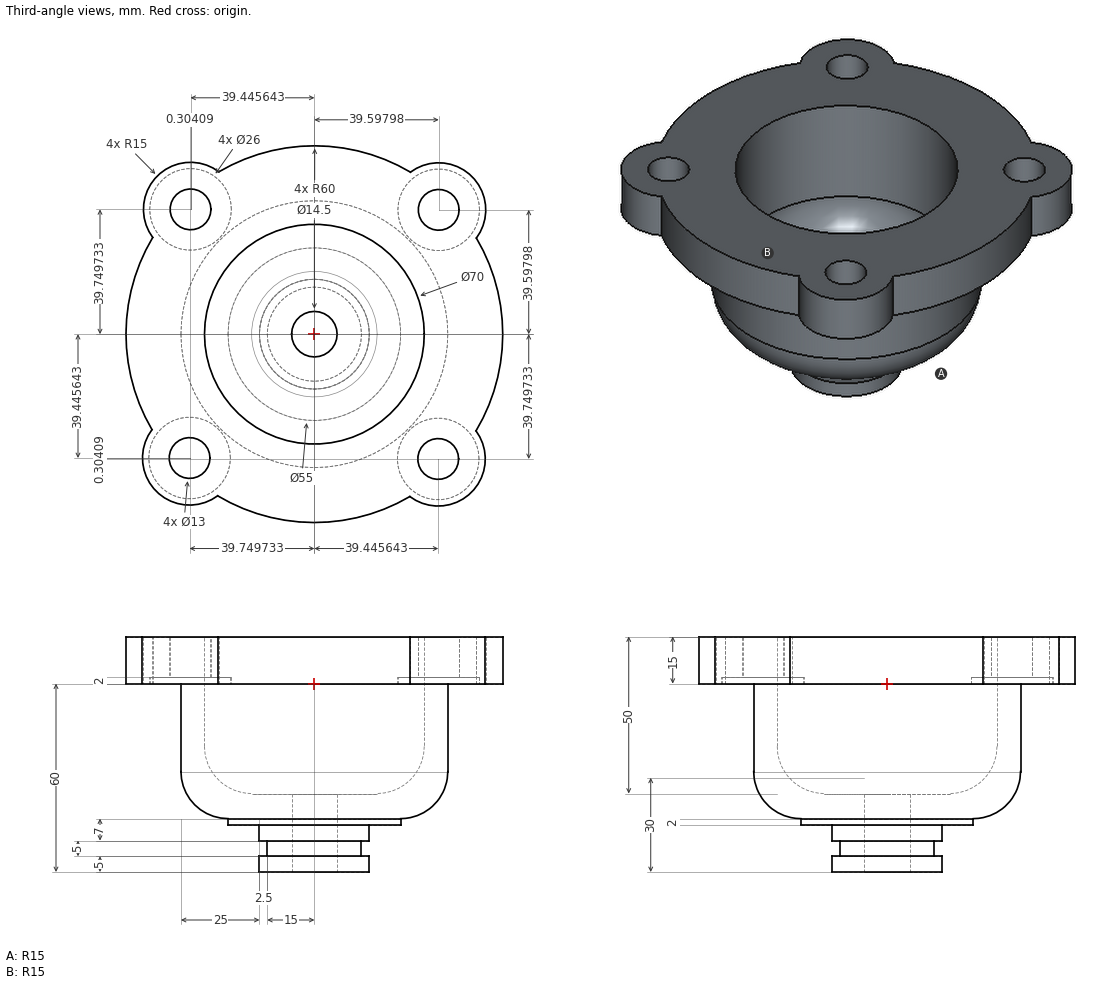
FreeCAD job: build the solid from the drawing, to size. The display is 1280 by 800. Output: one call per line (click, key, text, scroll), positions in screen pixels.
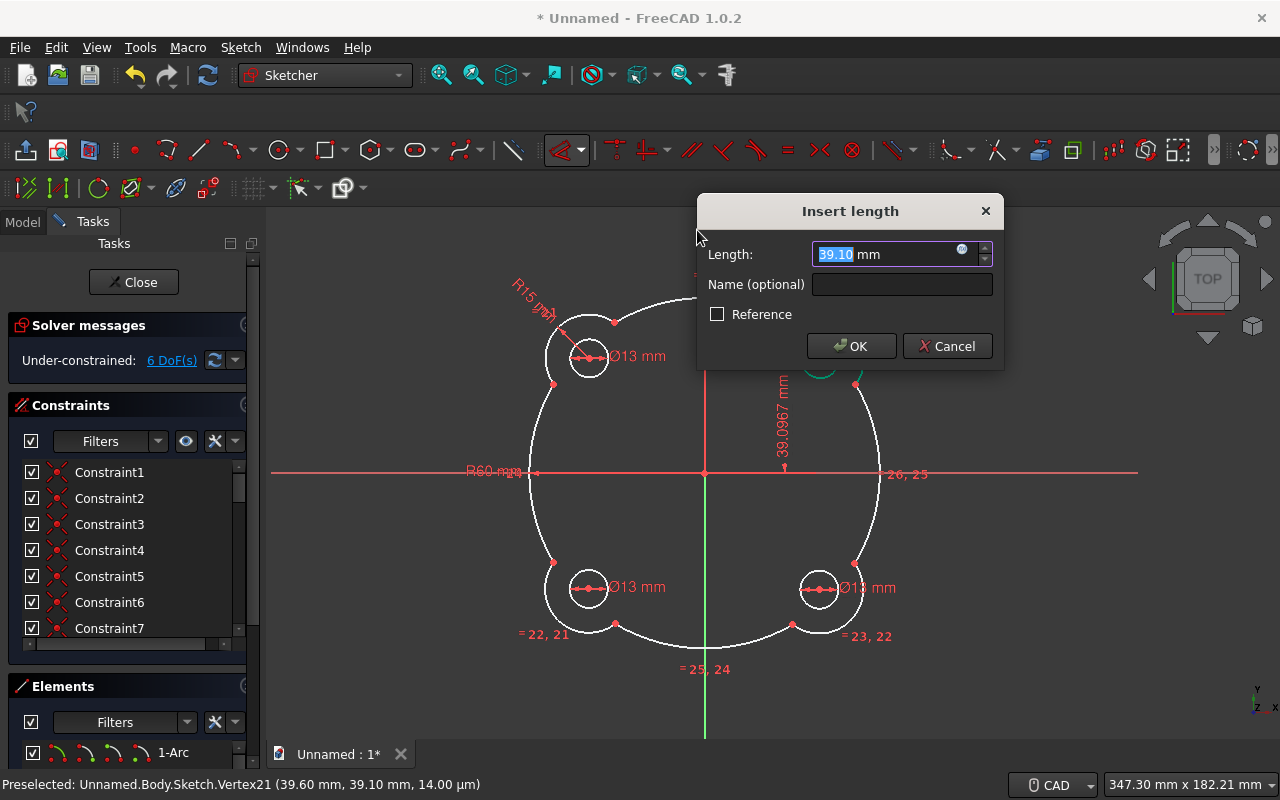
text(39.59798)
key(Return)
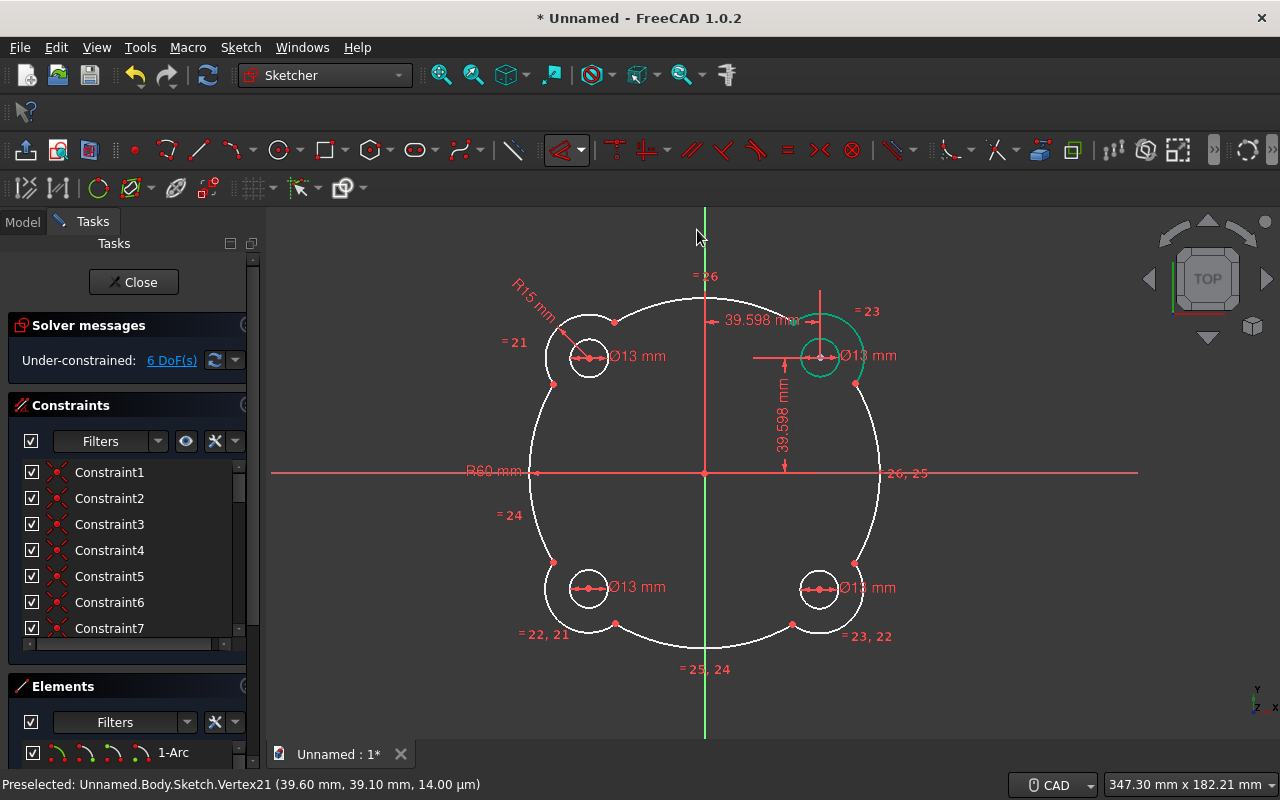
click(589, 589)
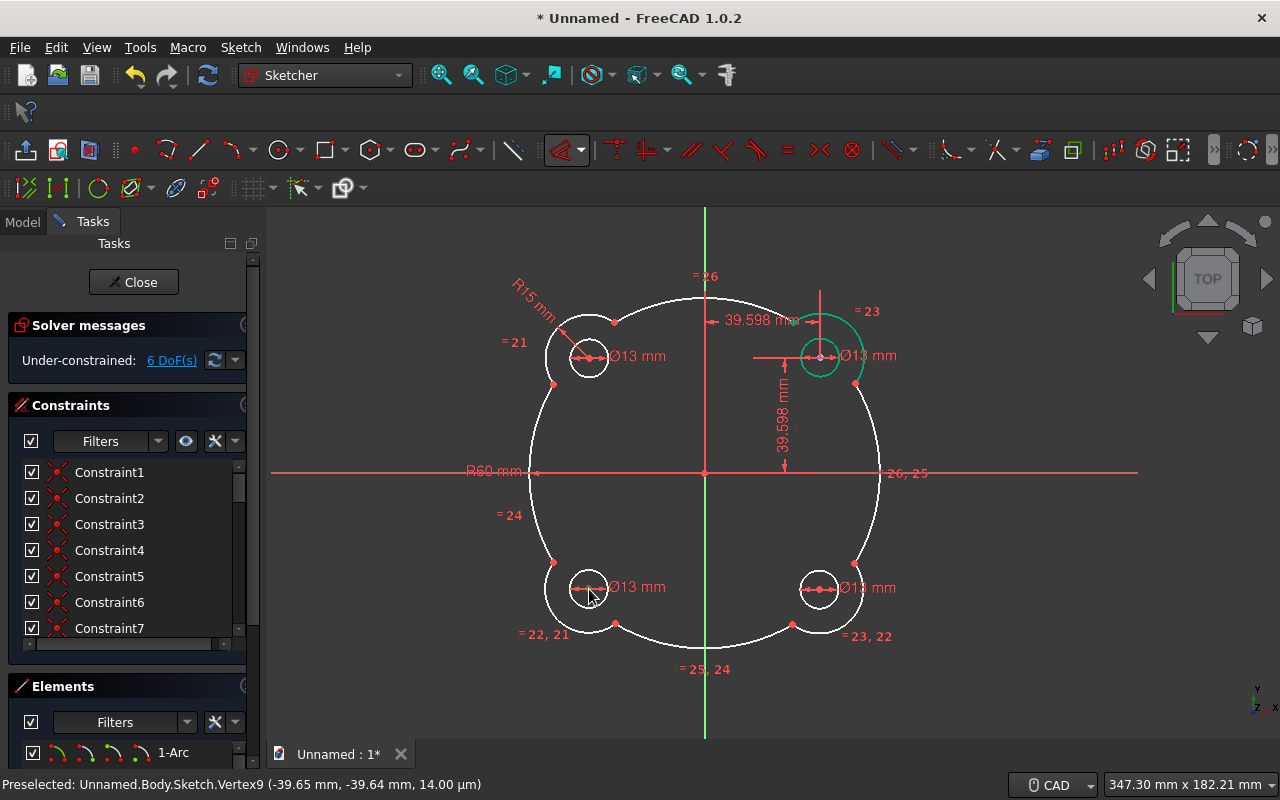
key(l)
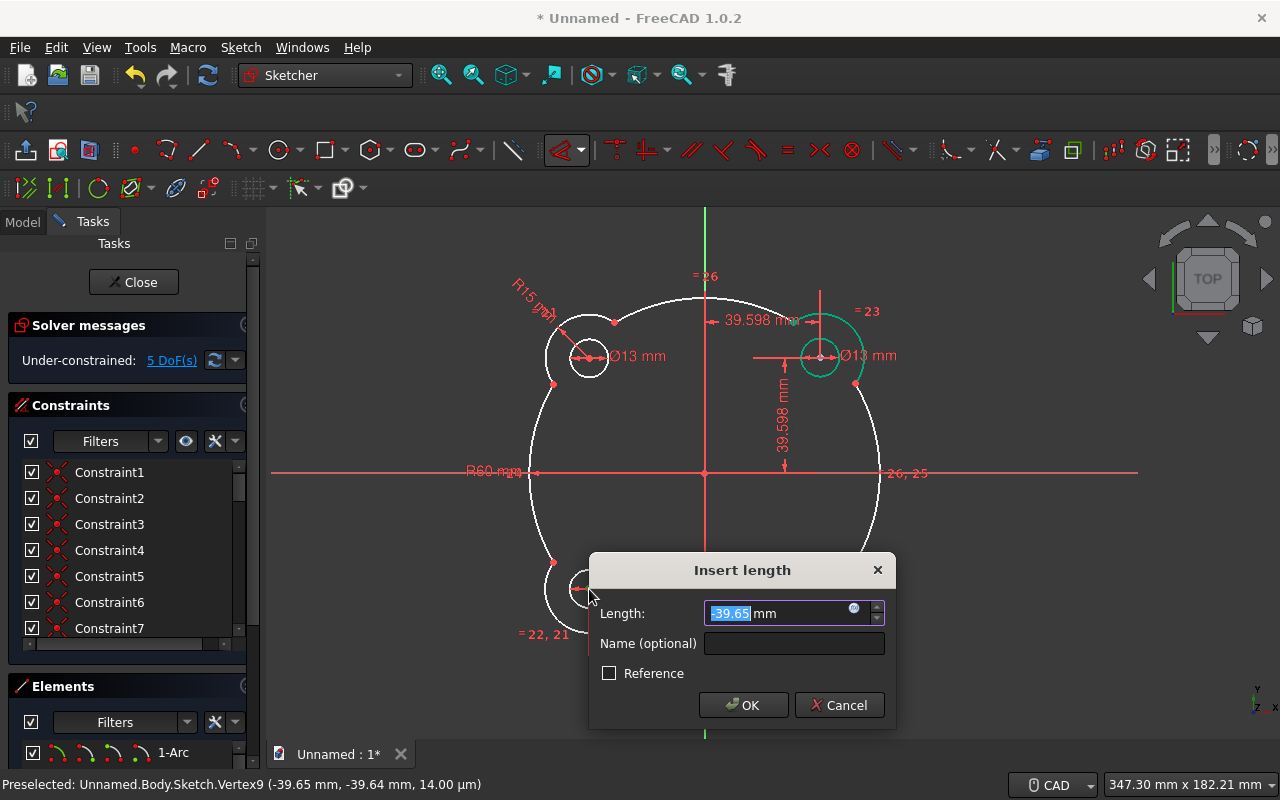
text(-39.749733)
key(Return)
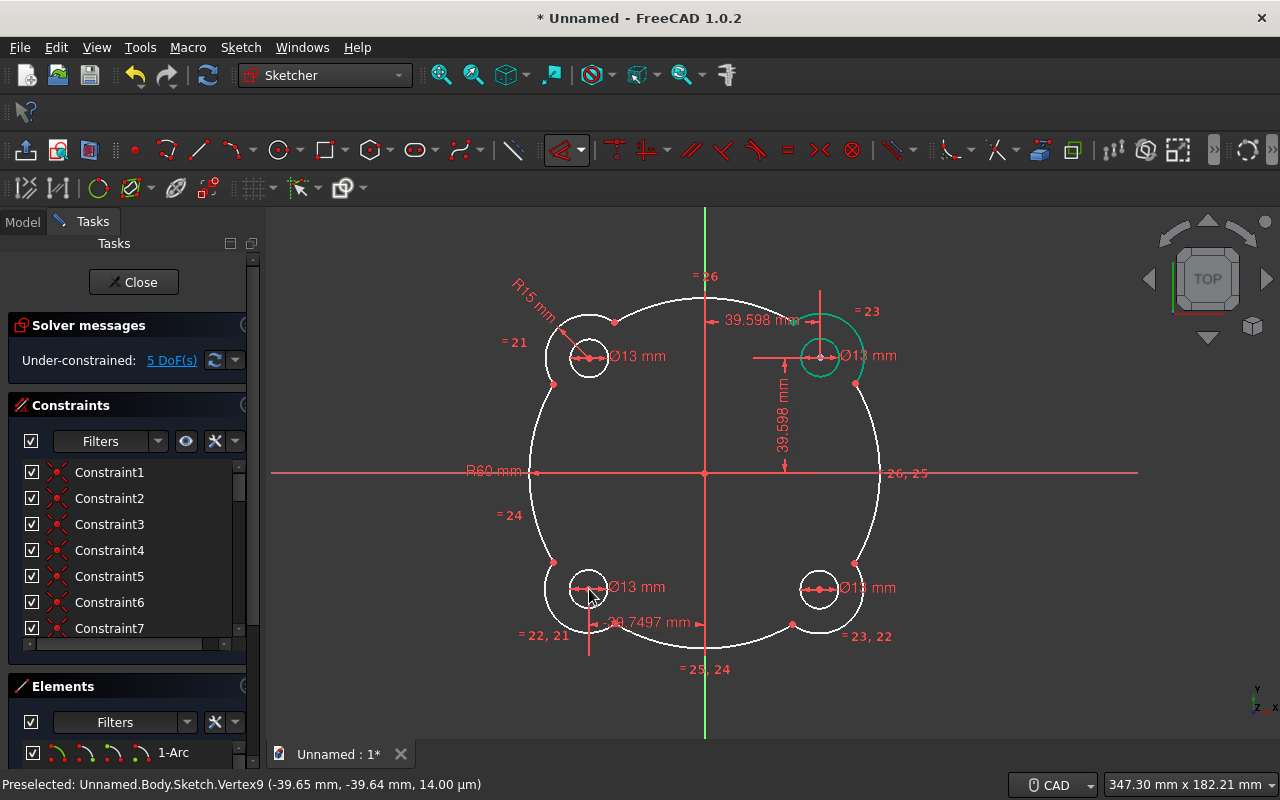
click(589, 589)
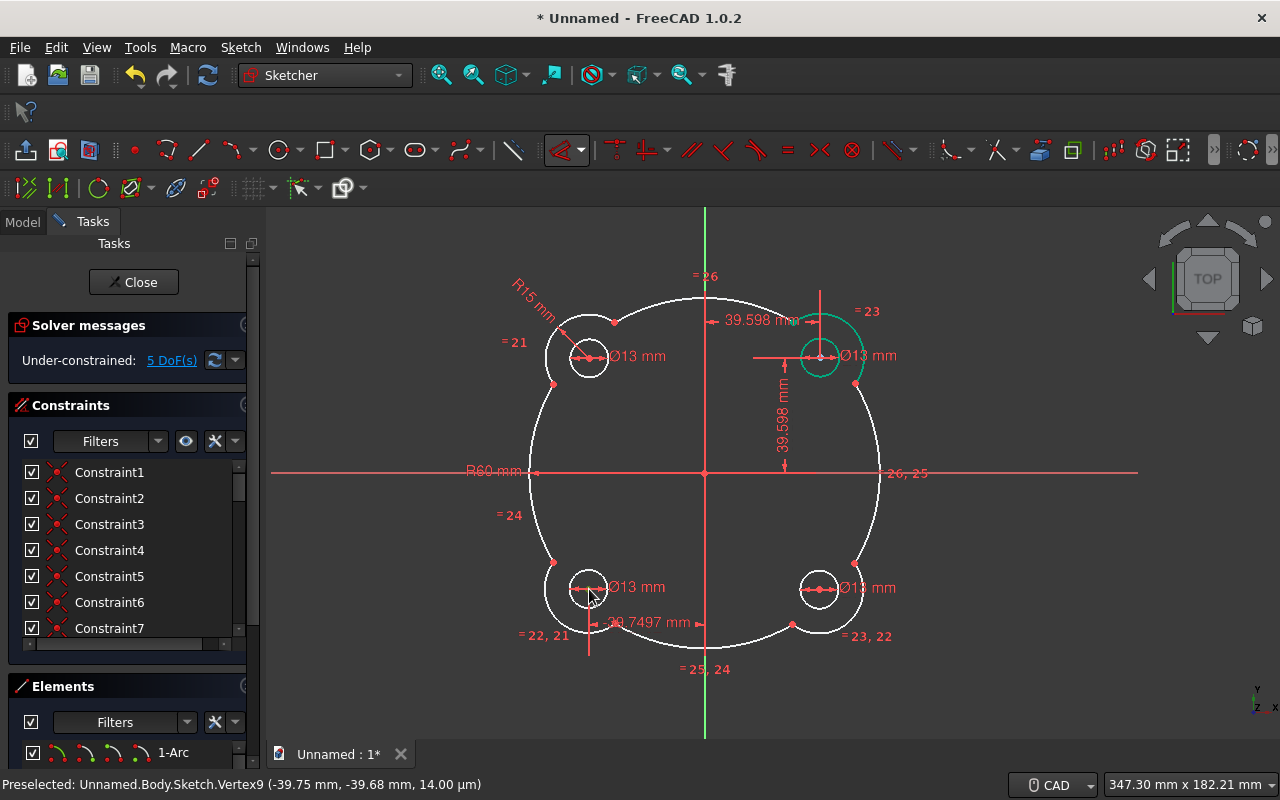
click(584, 150)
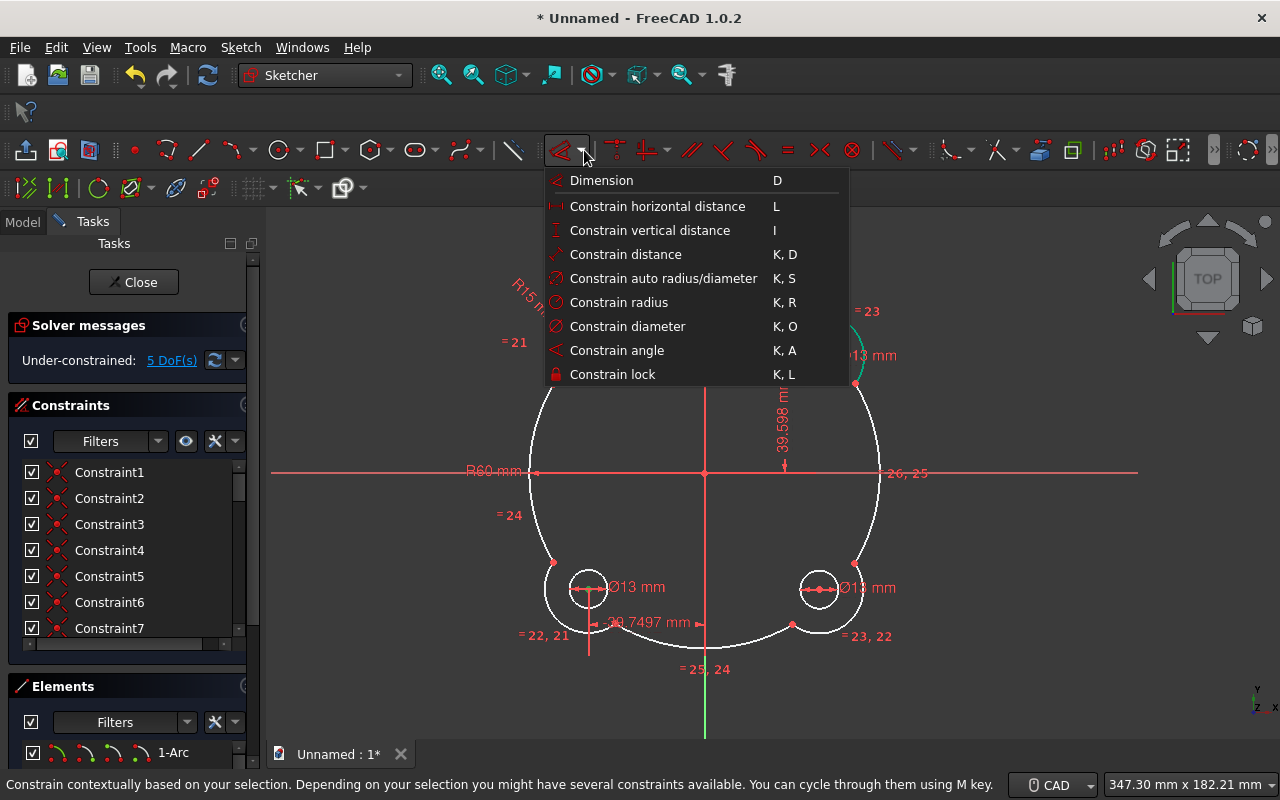
click(697, 230)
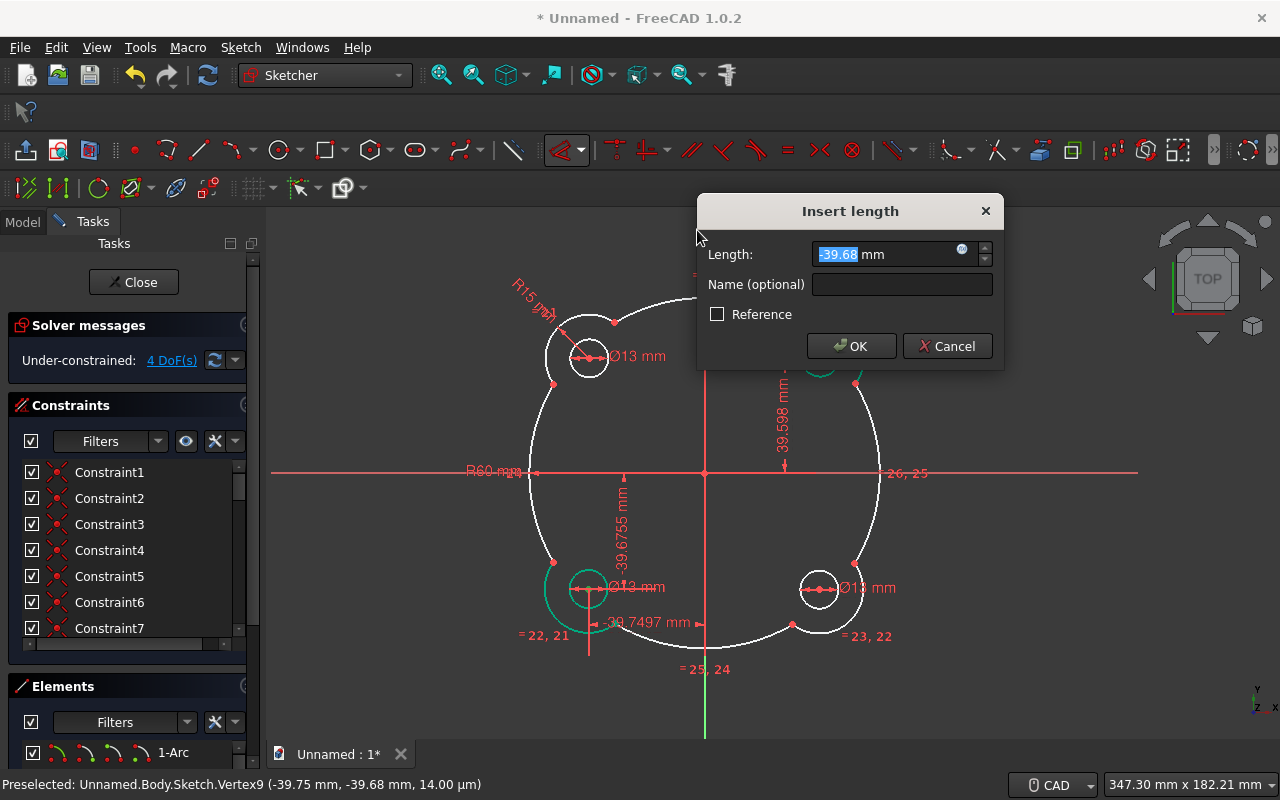
text(-39.445643)
key(Return)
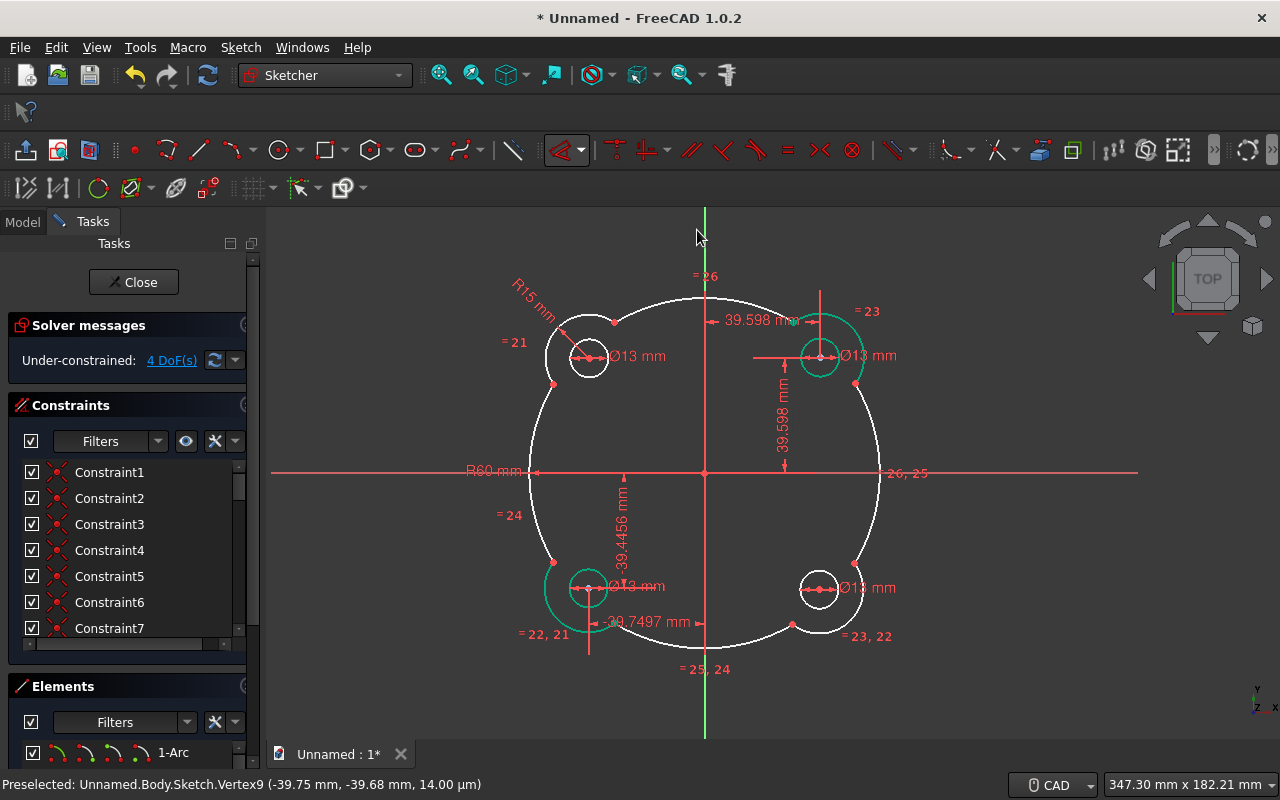
click(819, 590)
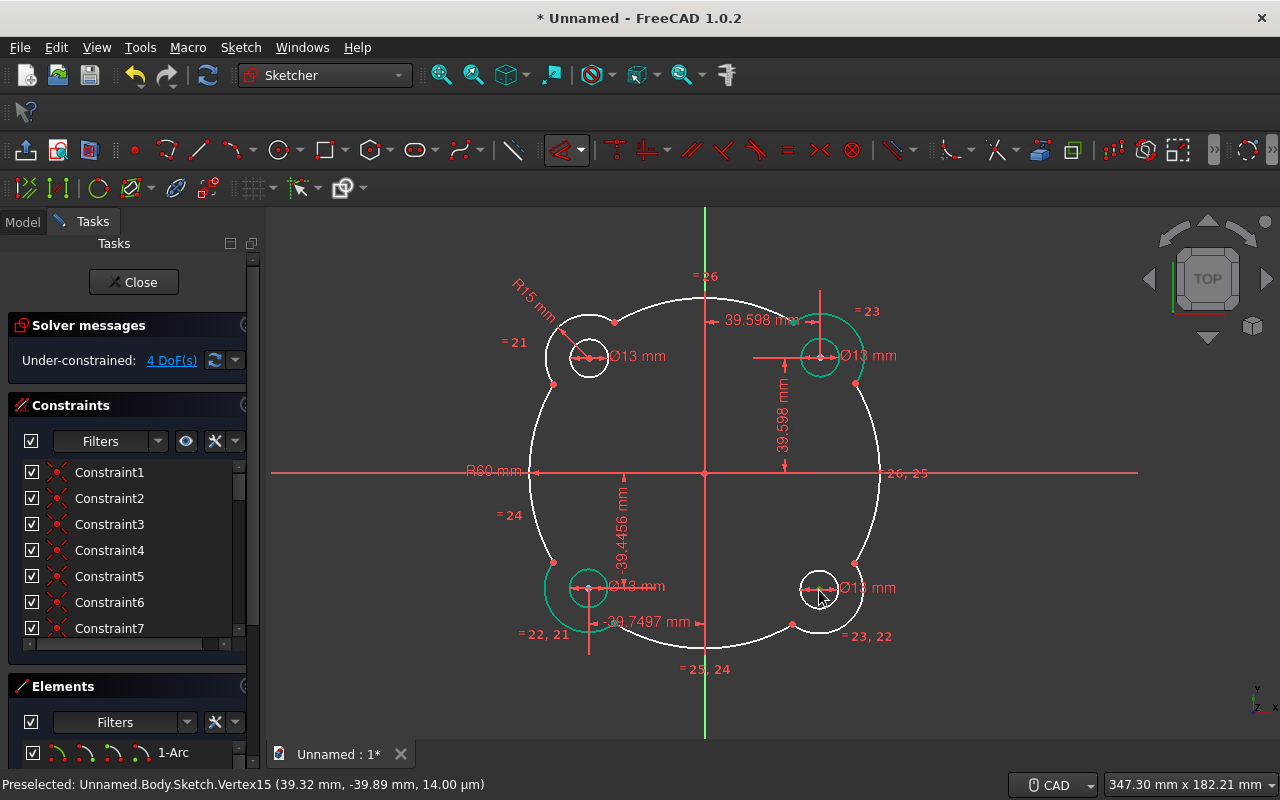
key(l)